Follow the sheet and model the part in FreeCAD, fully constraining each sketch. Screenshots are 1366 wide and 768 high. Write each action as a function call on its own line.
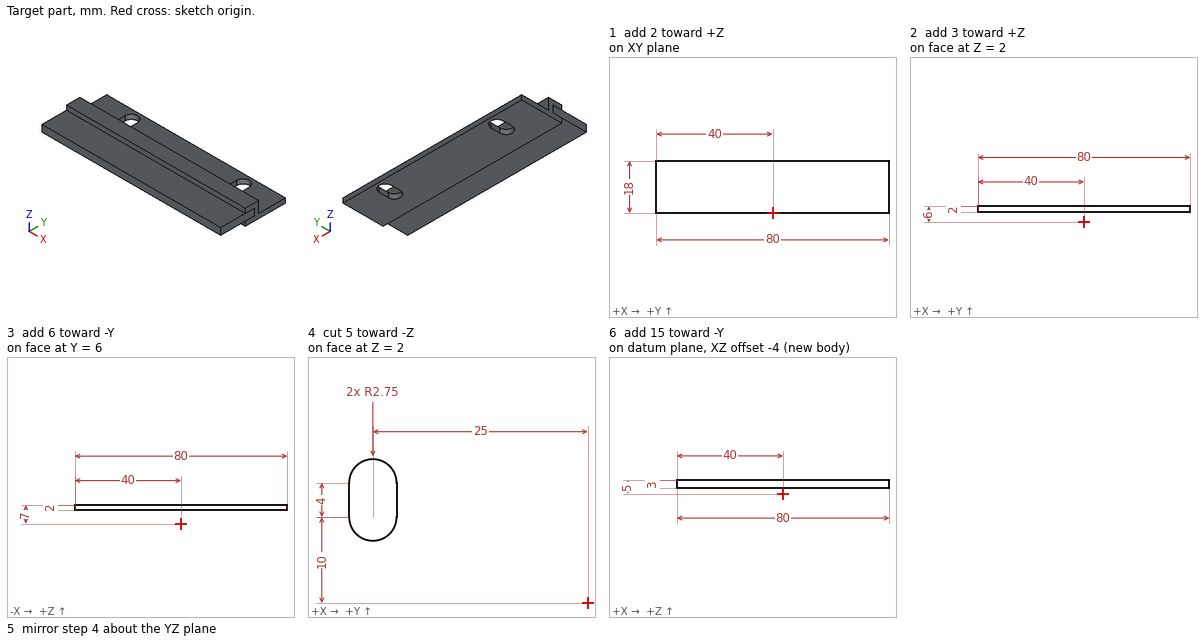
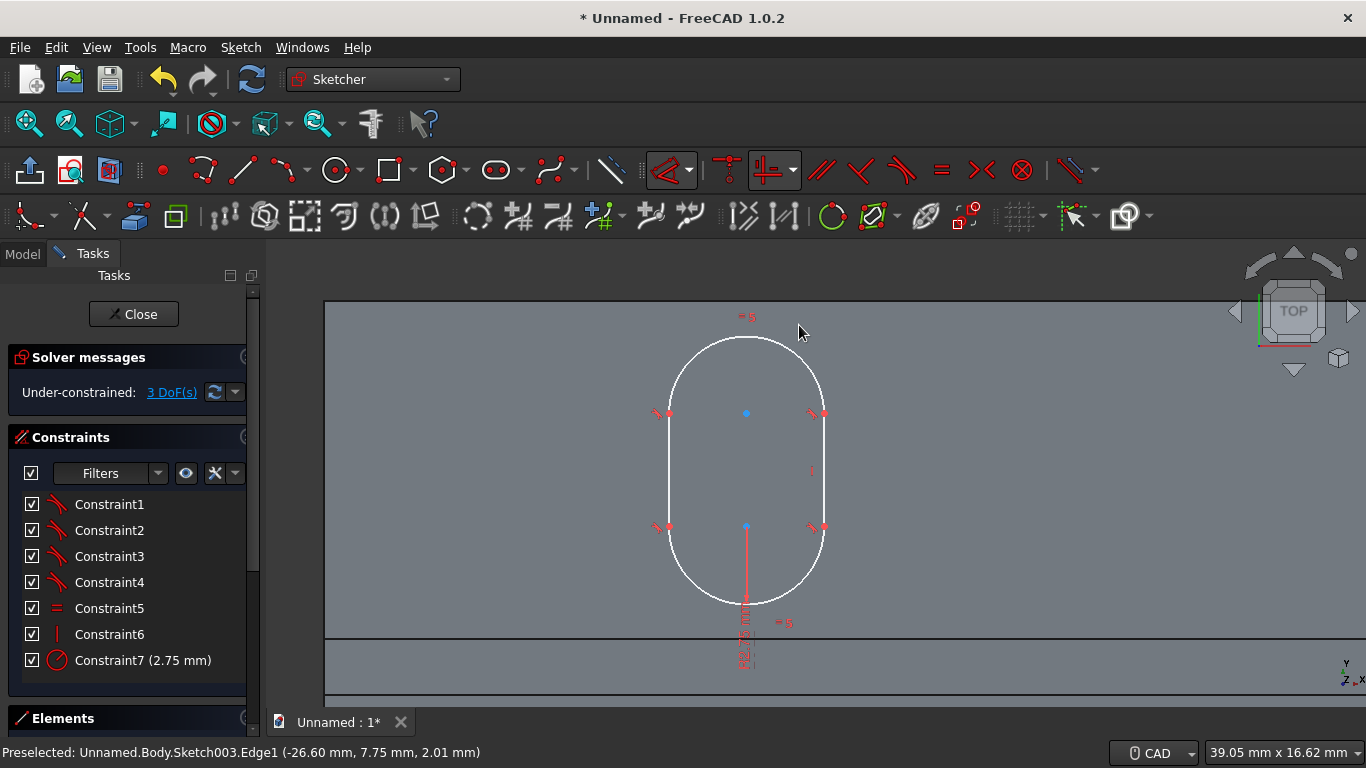
click(669, 493)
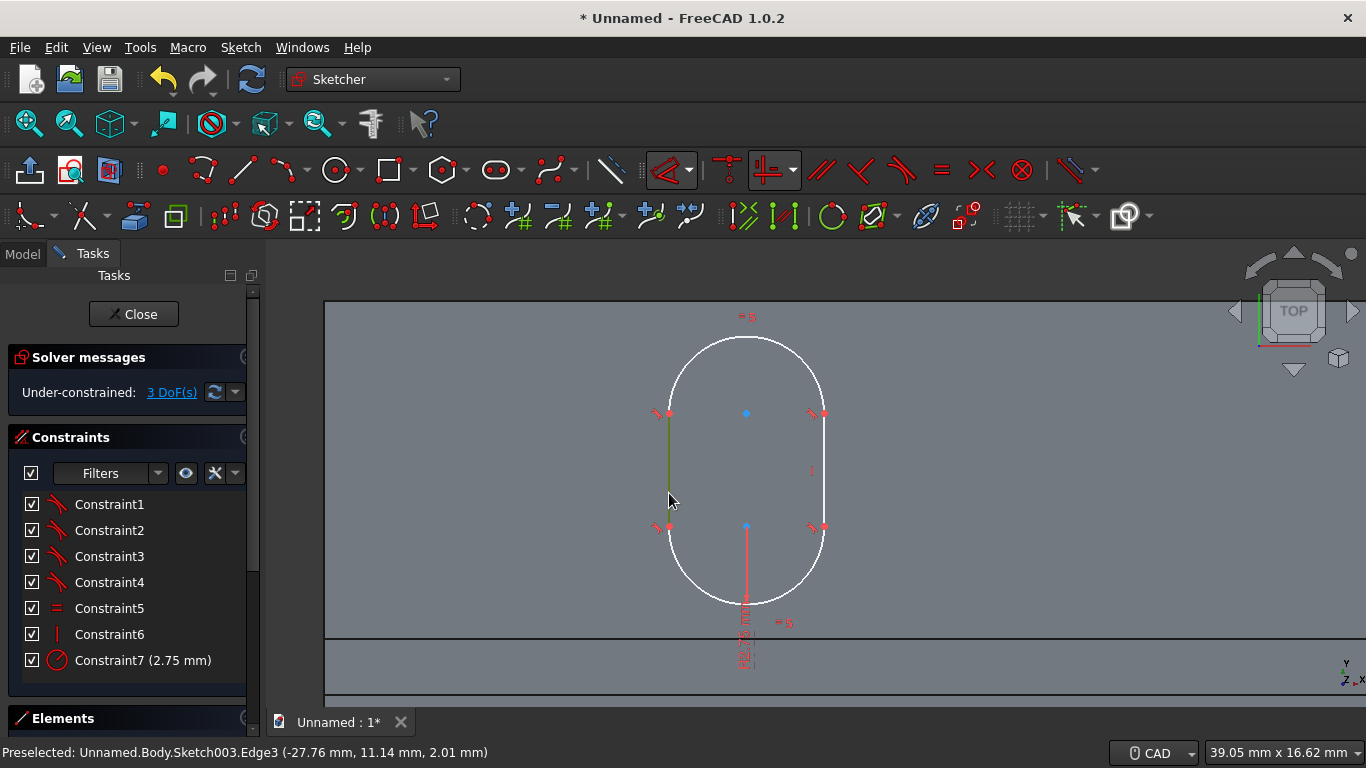
key(i)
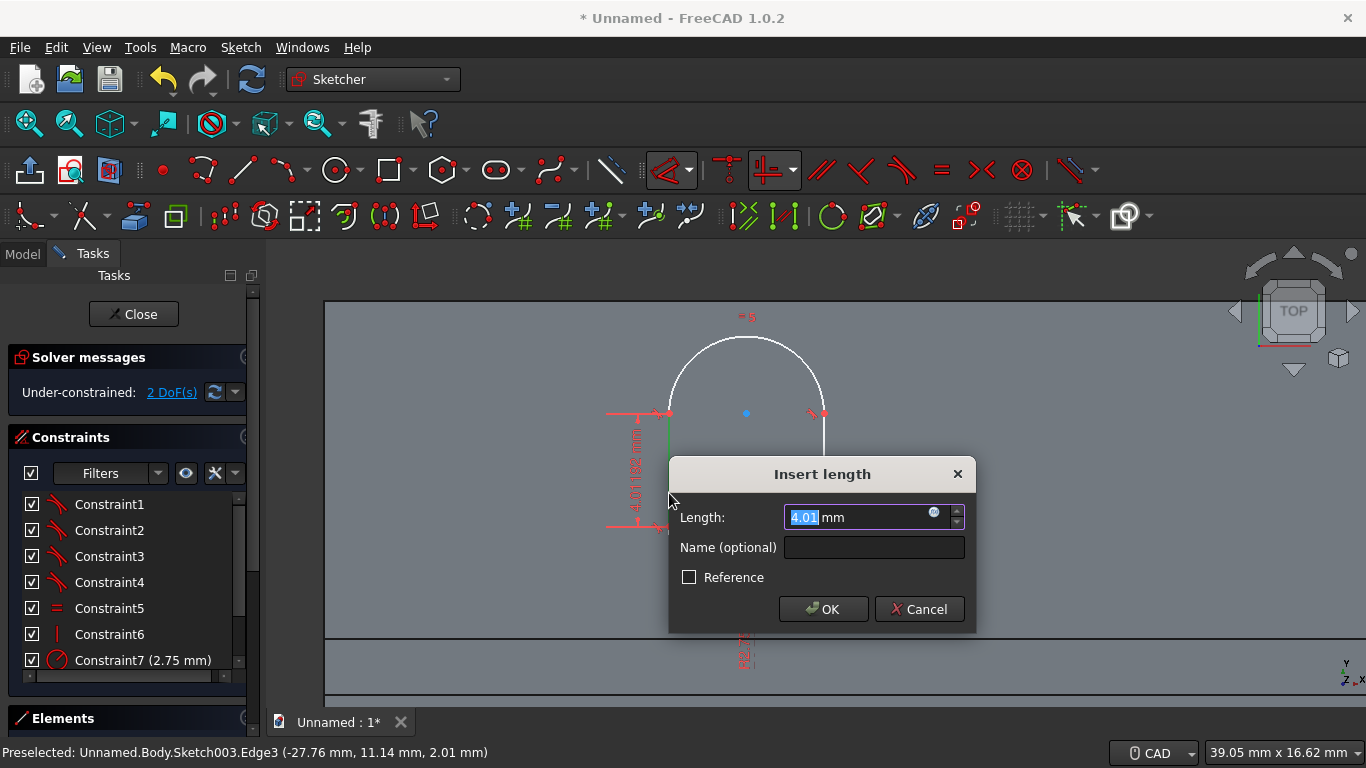
text(4)
key(Return)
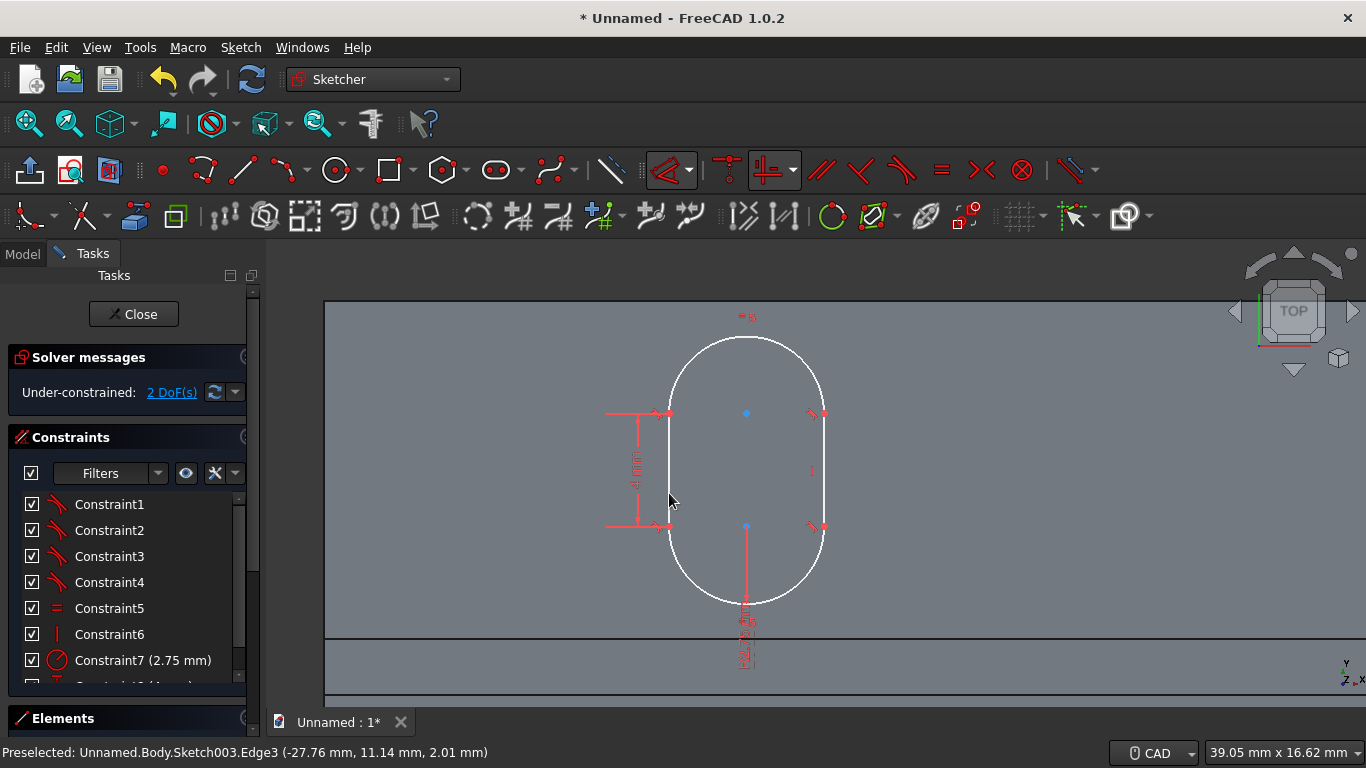
click(669, 527)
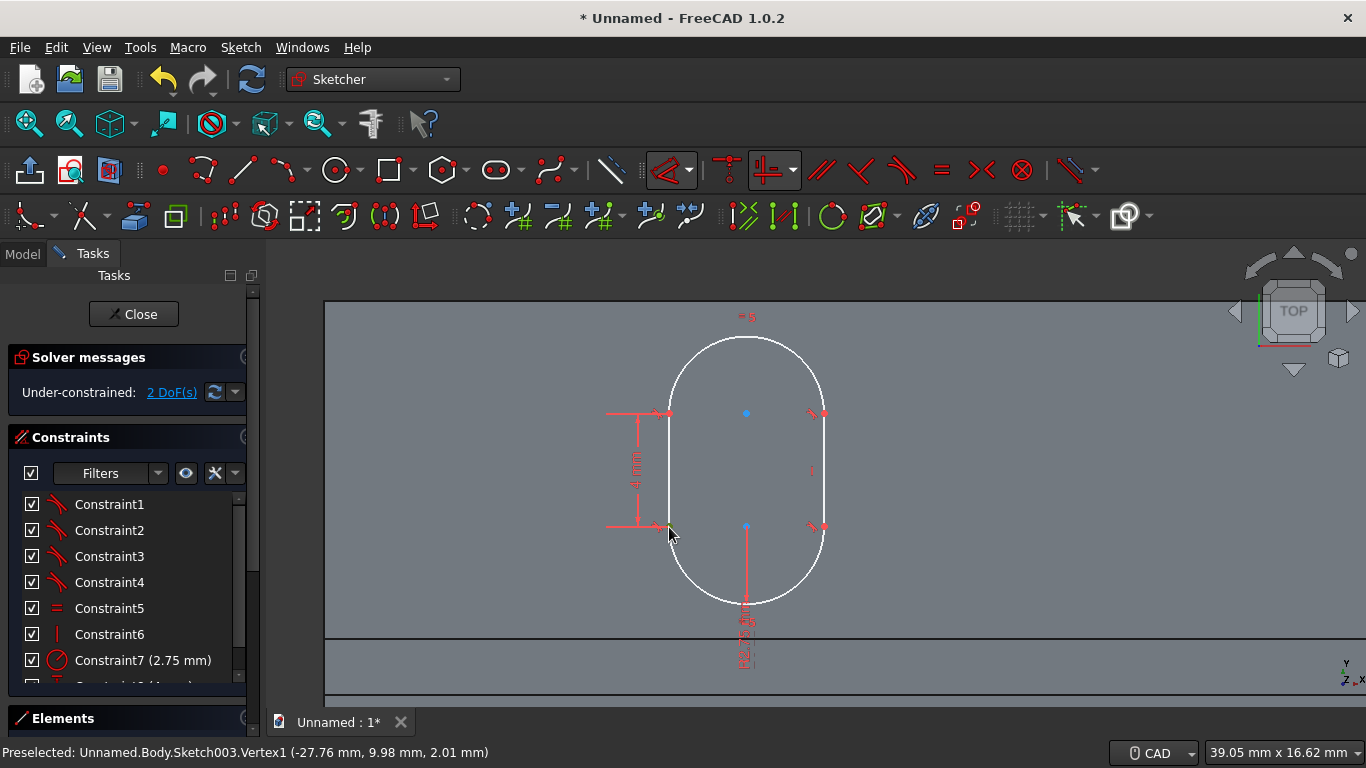
click(692, 170)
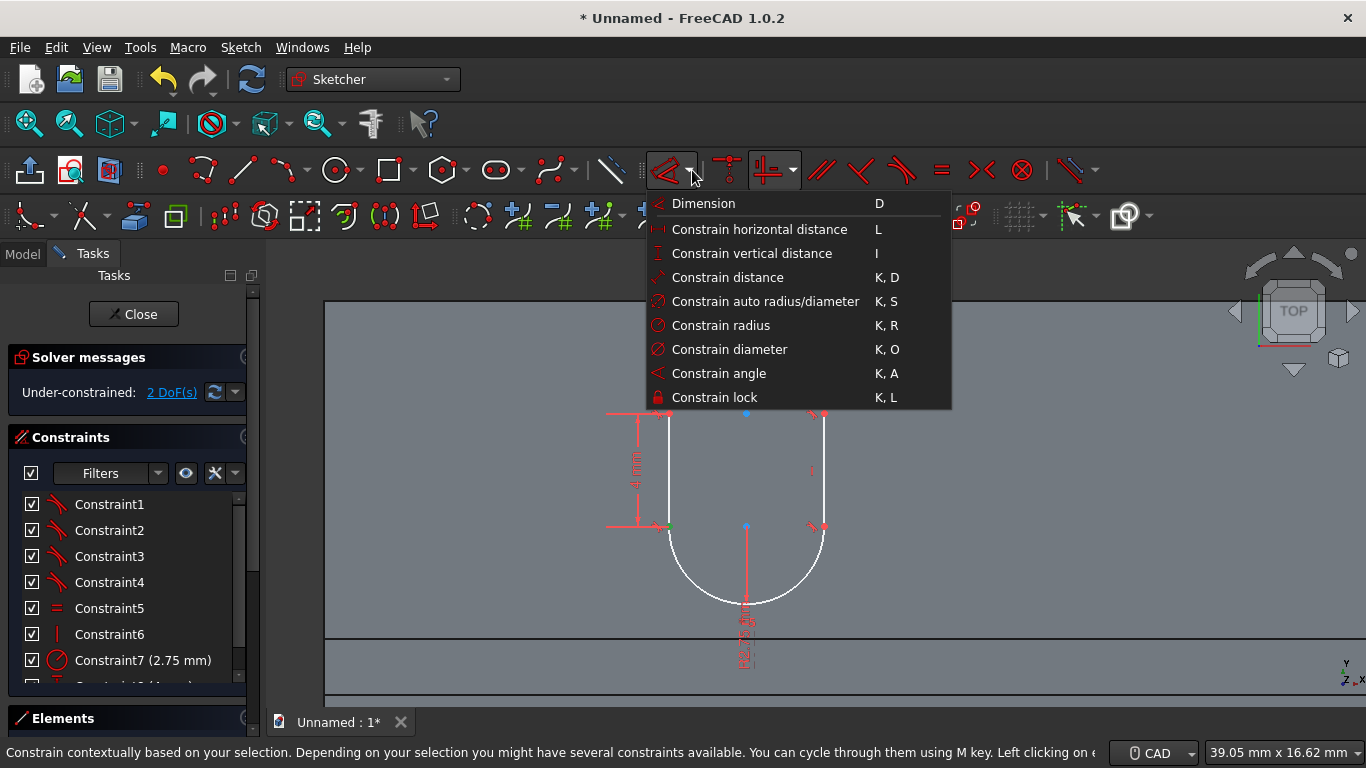
click(799, 253)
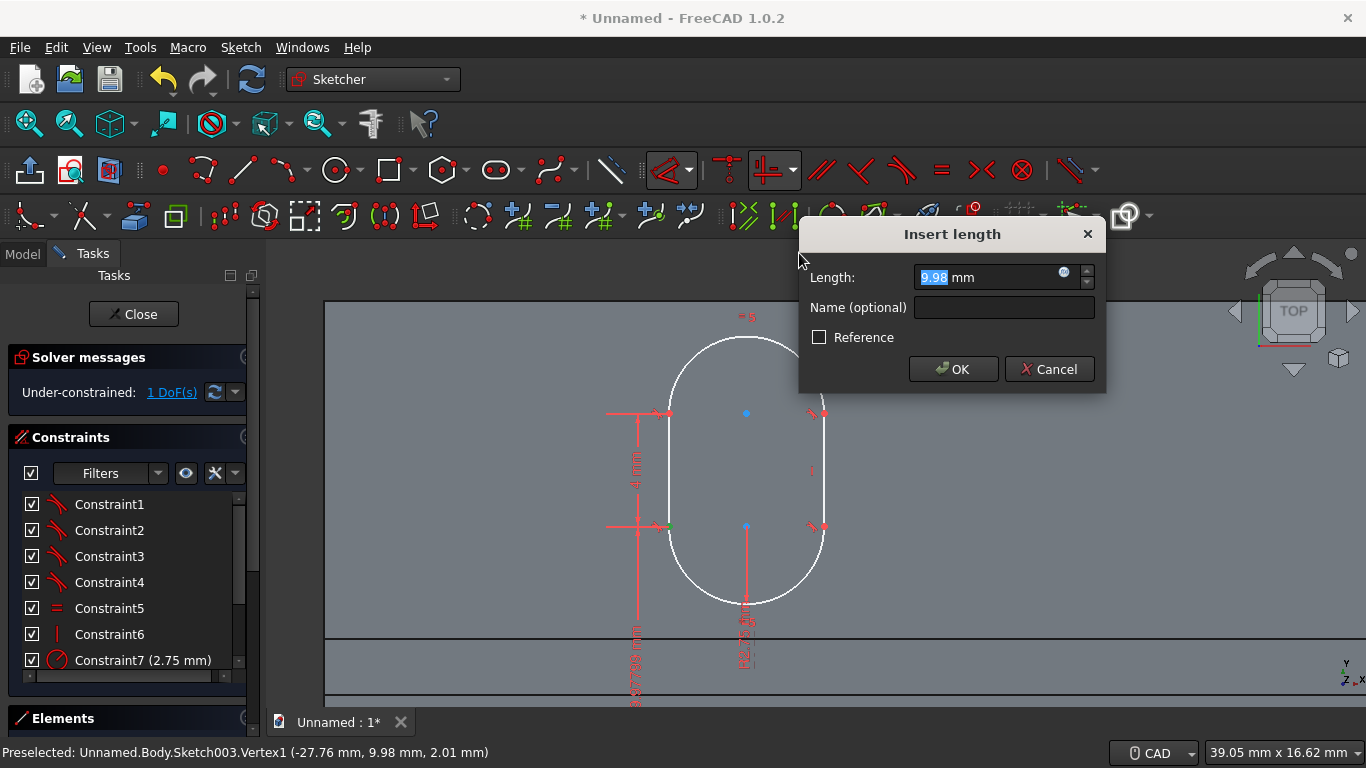
text(10)
key(Return)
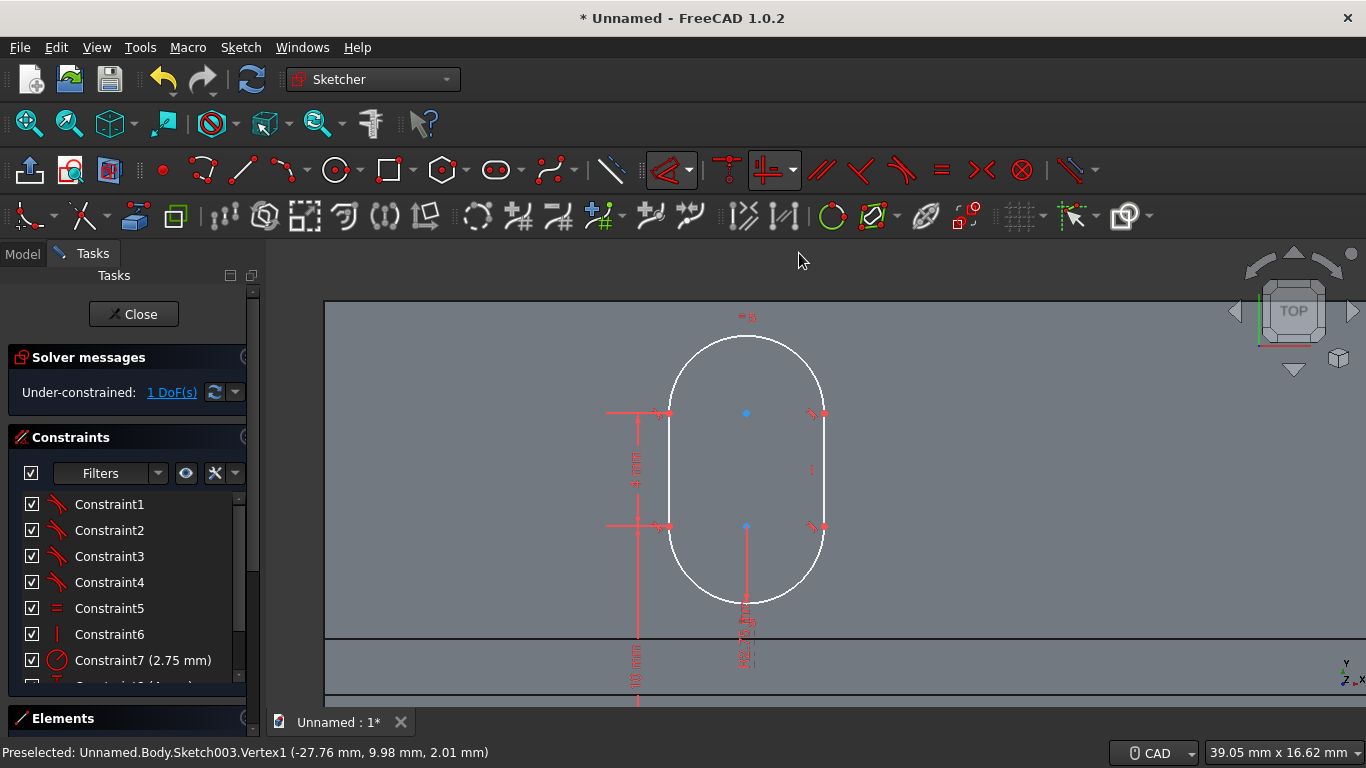
click(747, 526)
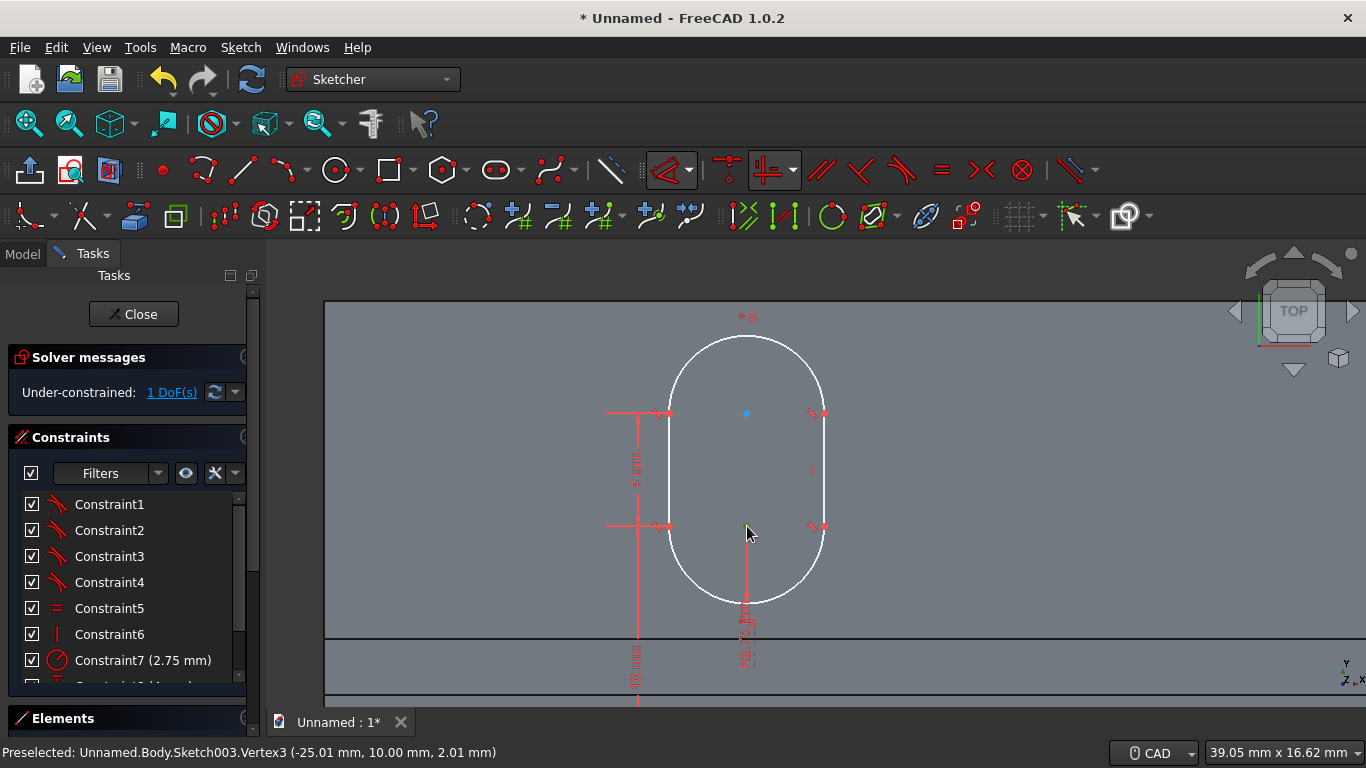
key(l)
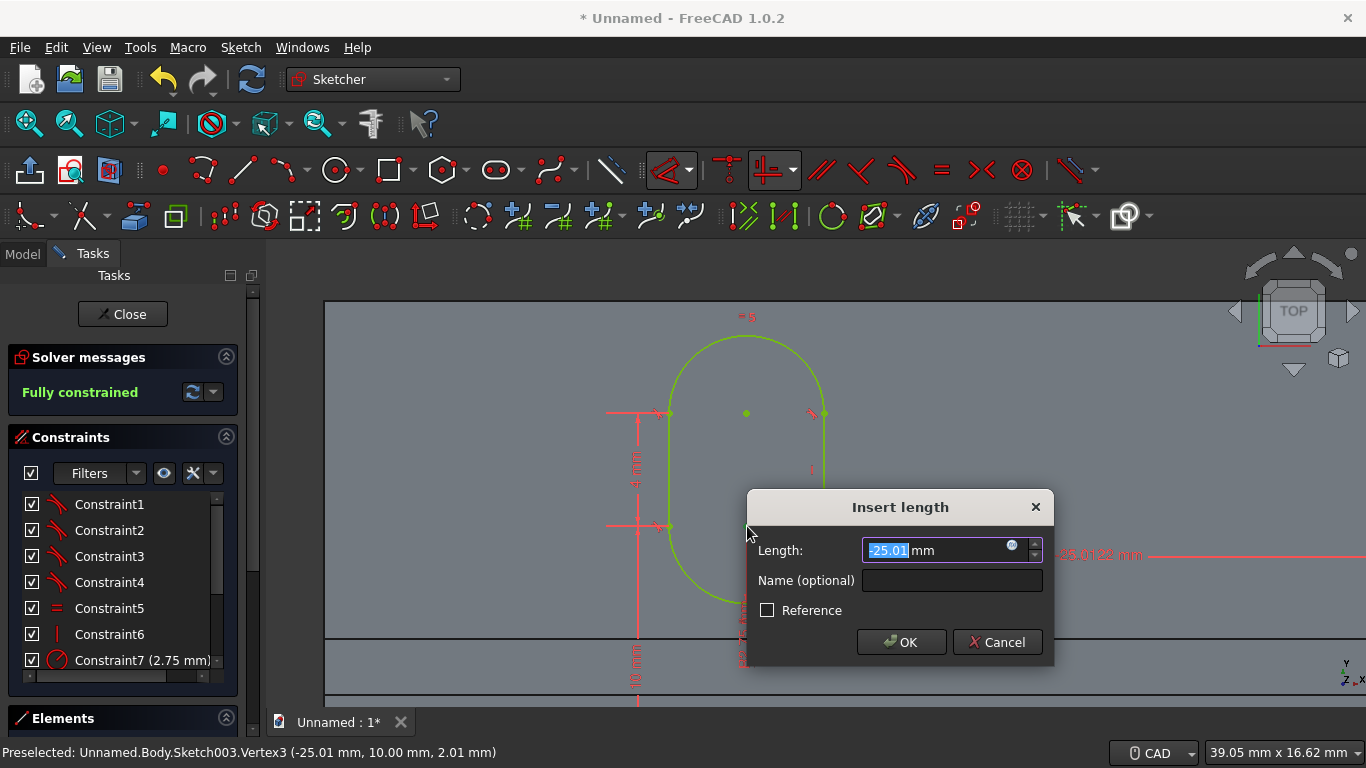
text(-25)
key(Return)